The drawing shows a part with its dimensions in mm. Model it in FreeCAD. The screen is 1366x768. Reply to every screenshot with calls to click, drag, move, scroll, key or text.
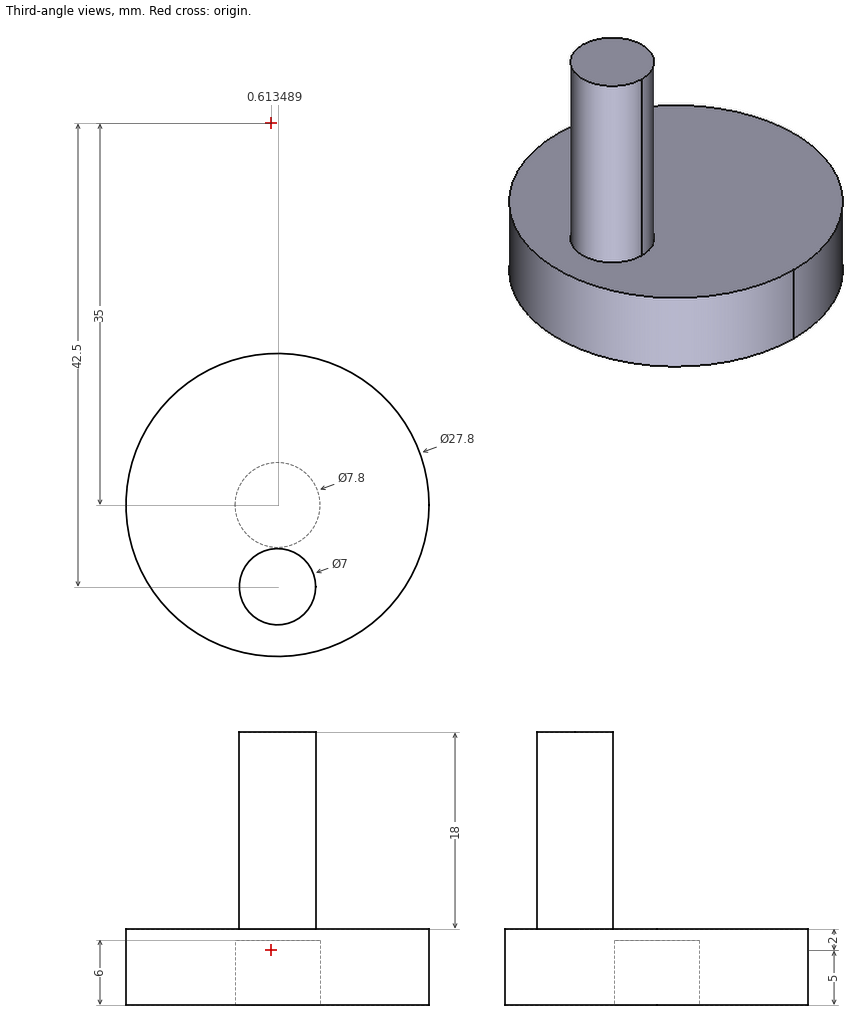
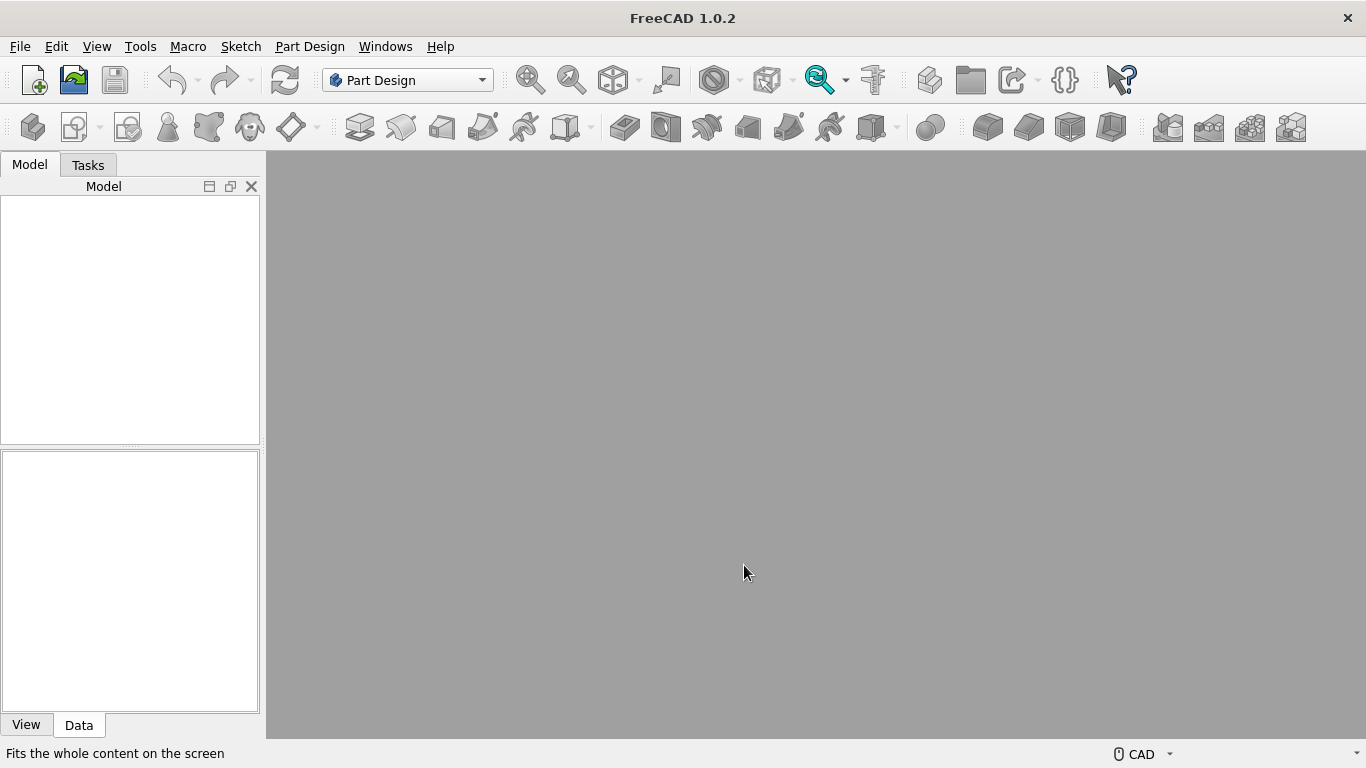
click(33, 80)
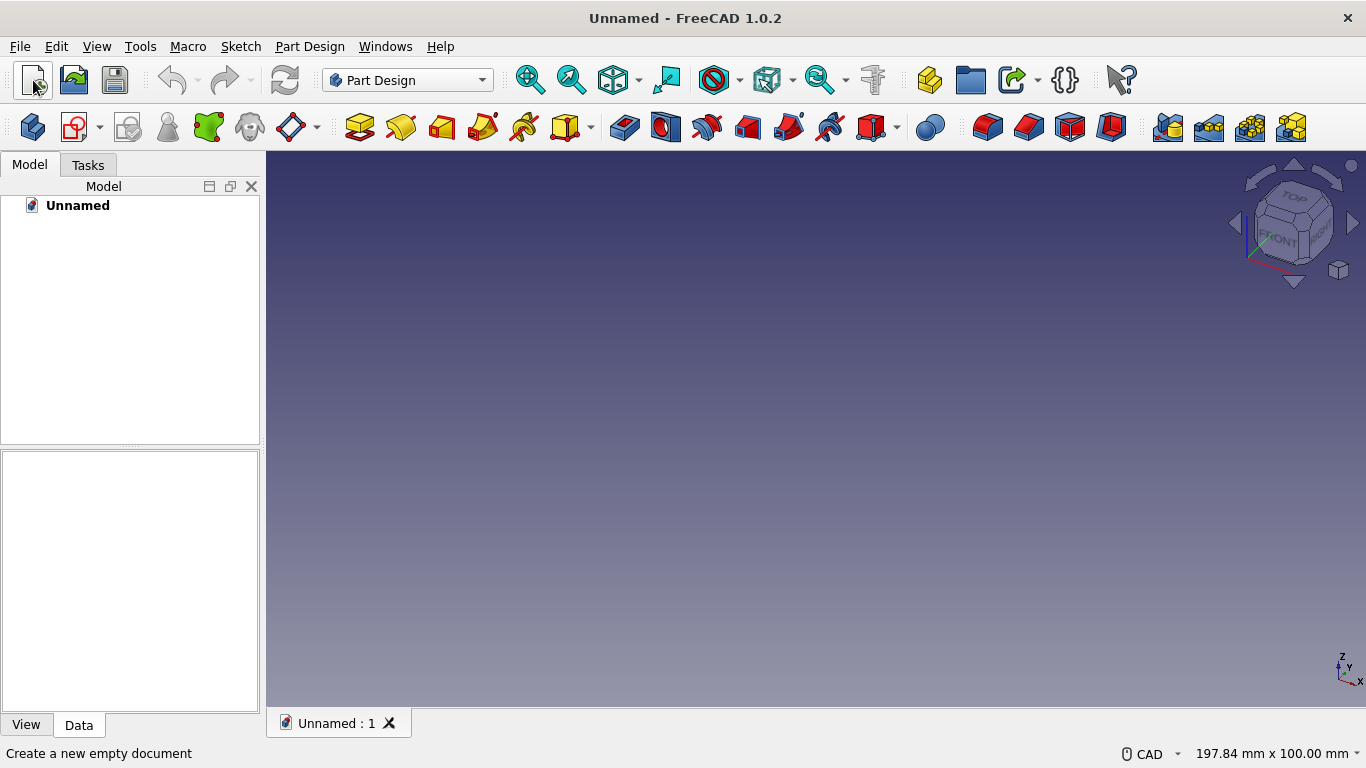
click(74, 128)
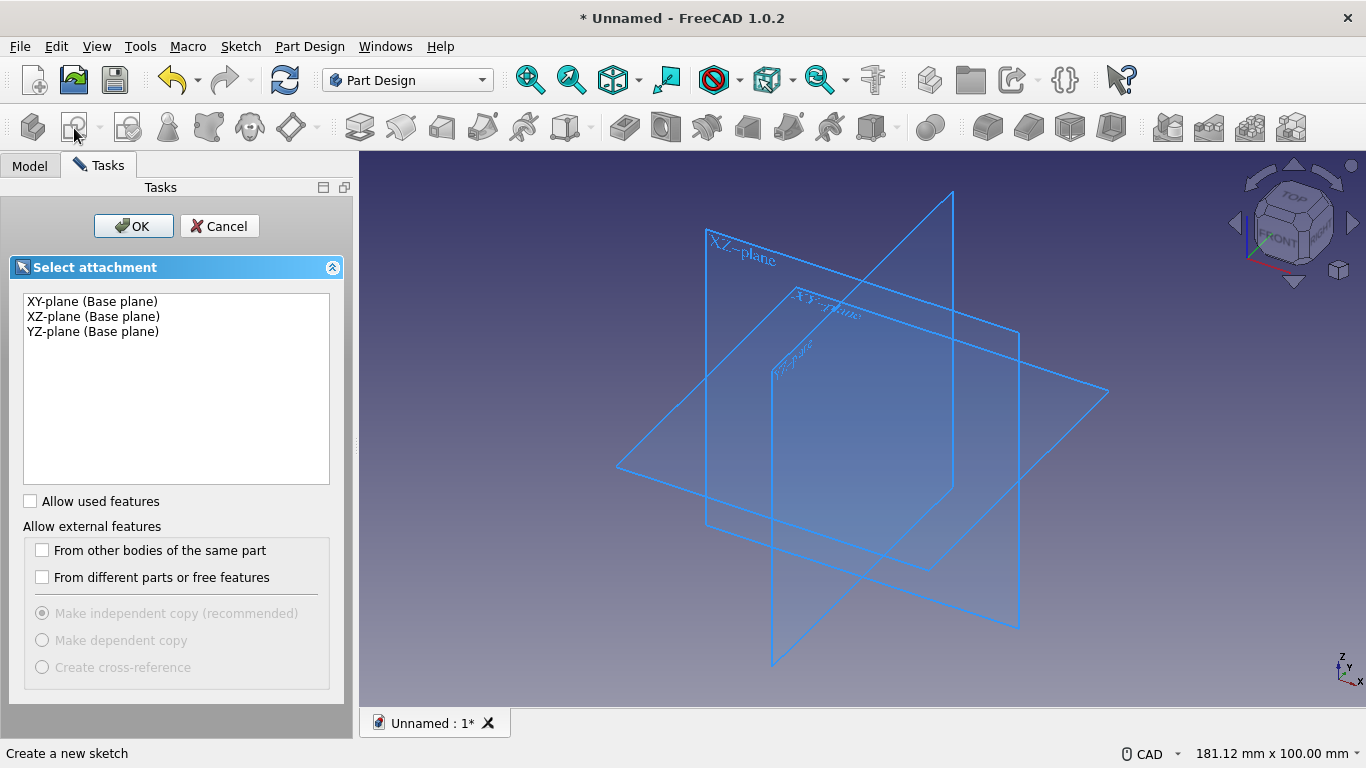
click(84, 302)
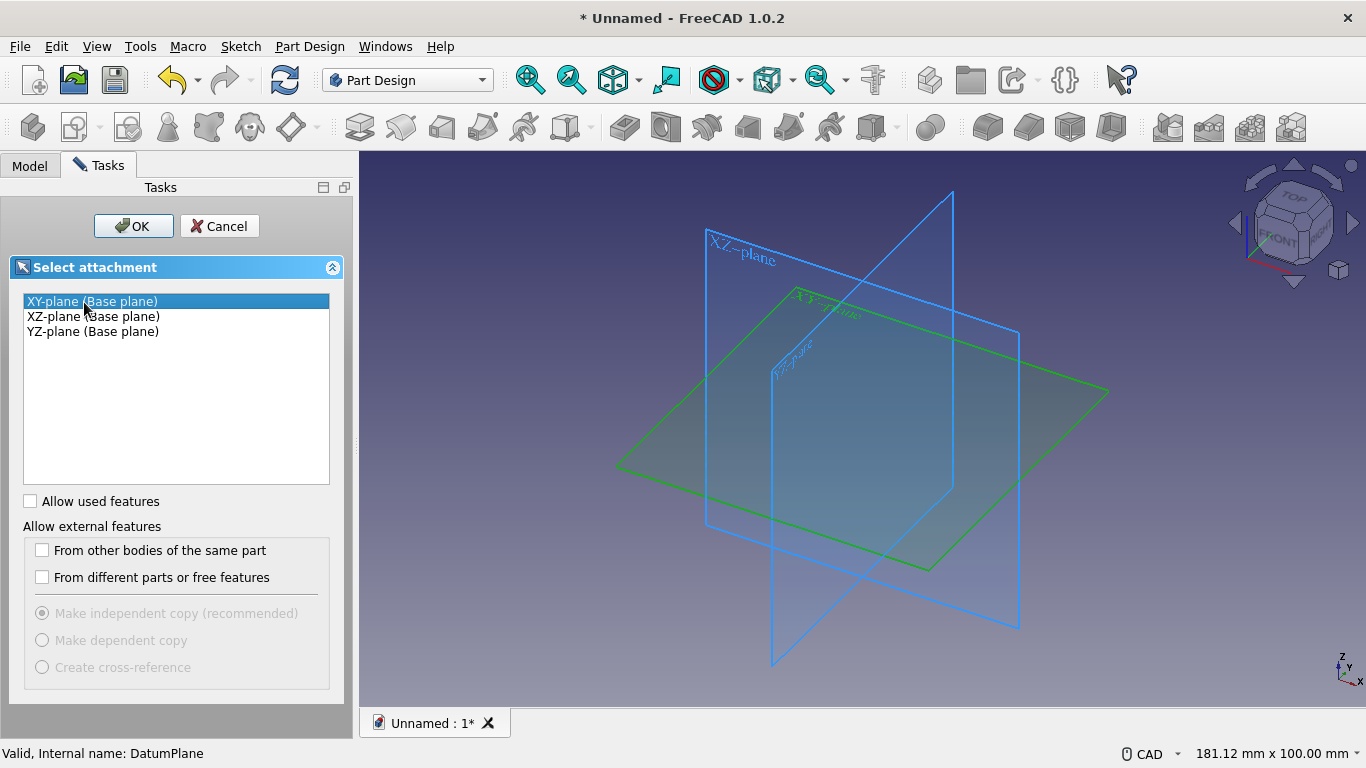
click(134, 226)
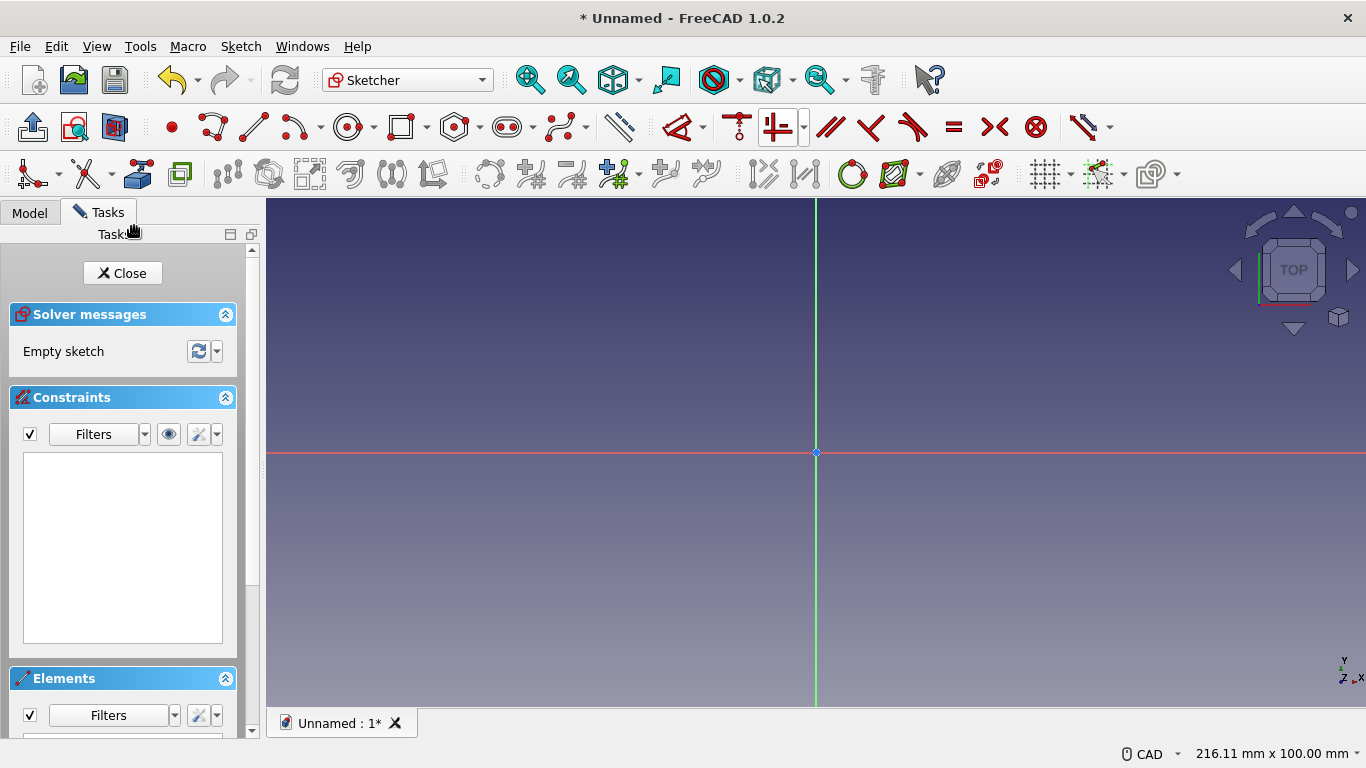
scroll(424, 226, down, 1)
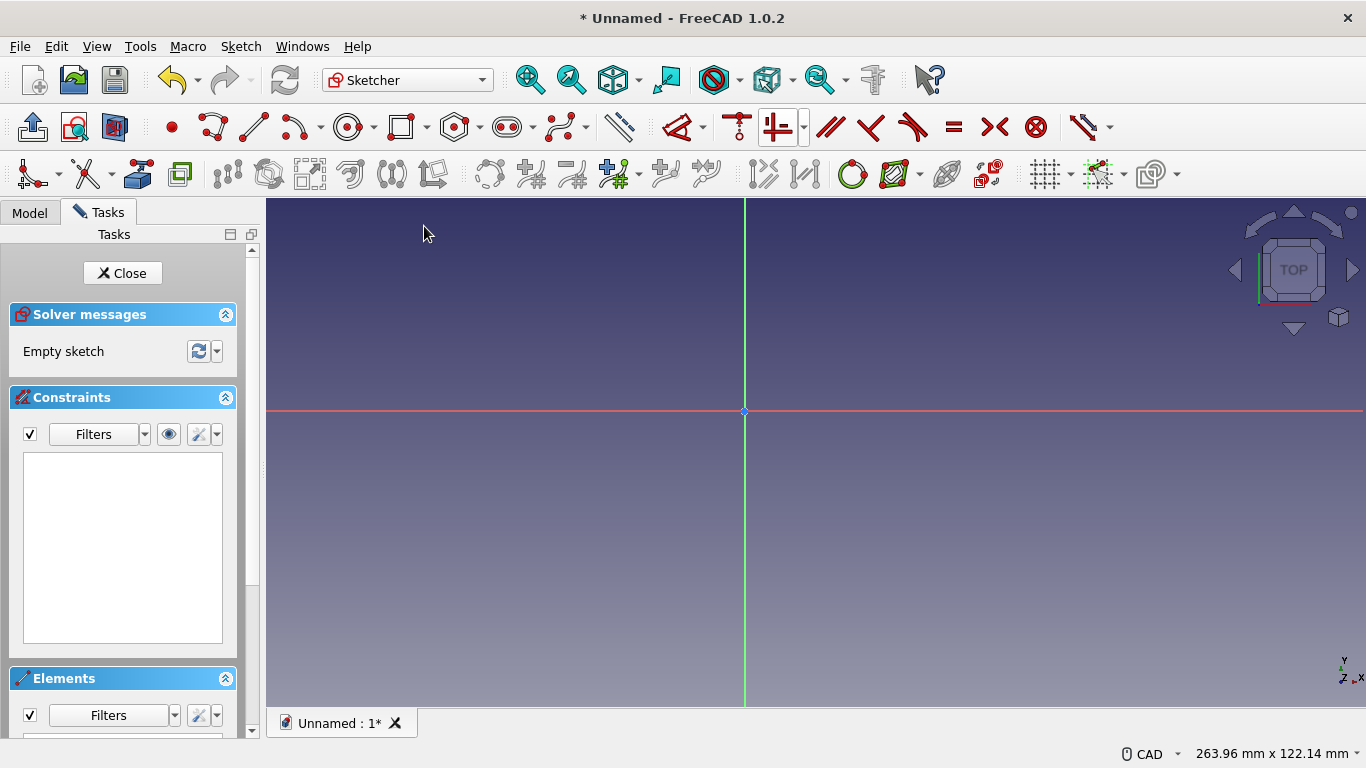
scroll(748, 637, up, 2)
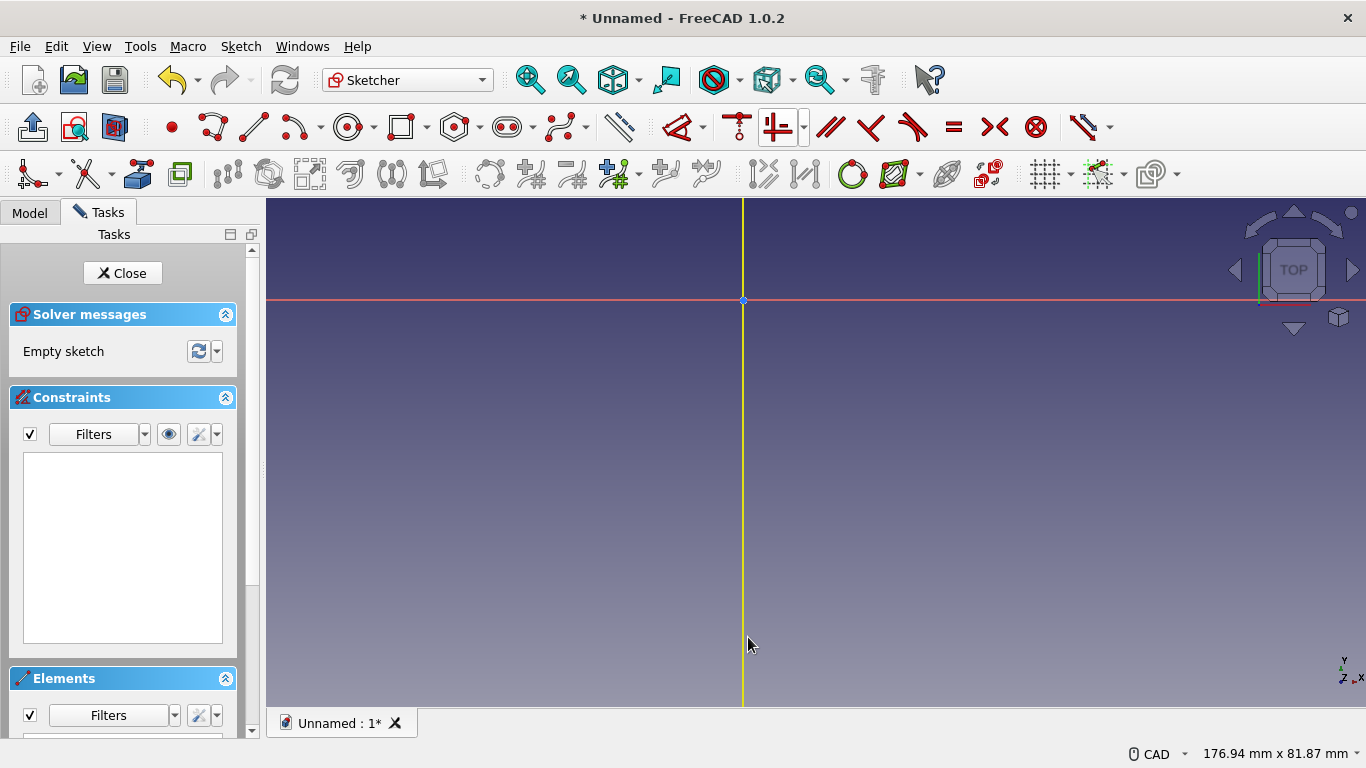
click(348, 128)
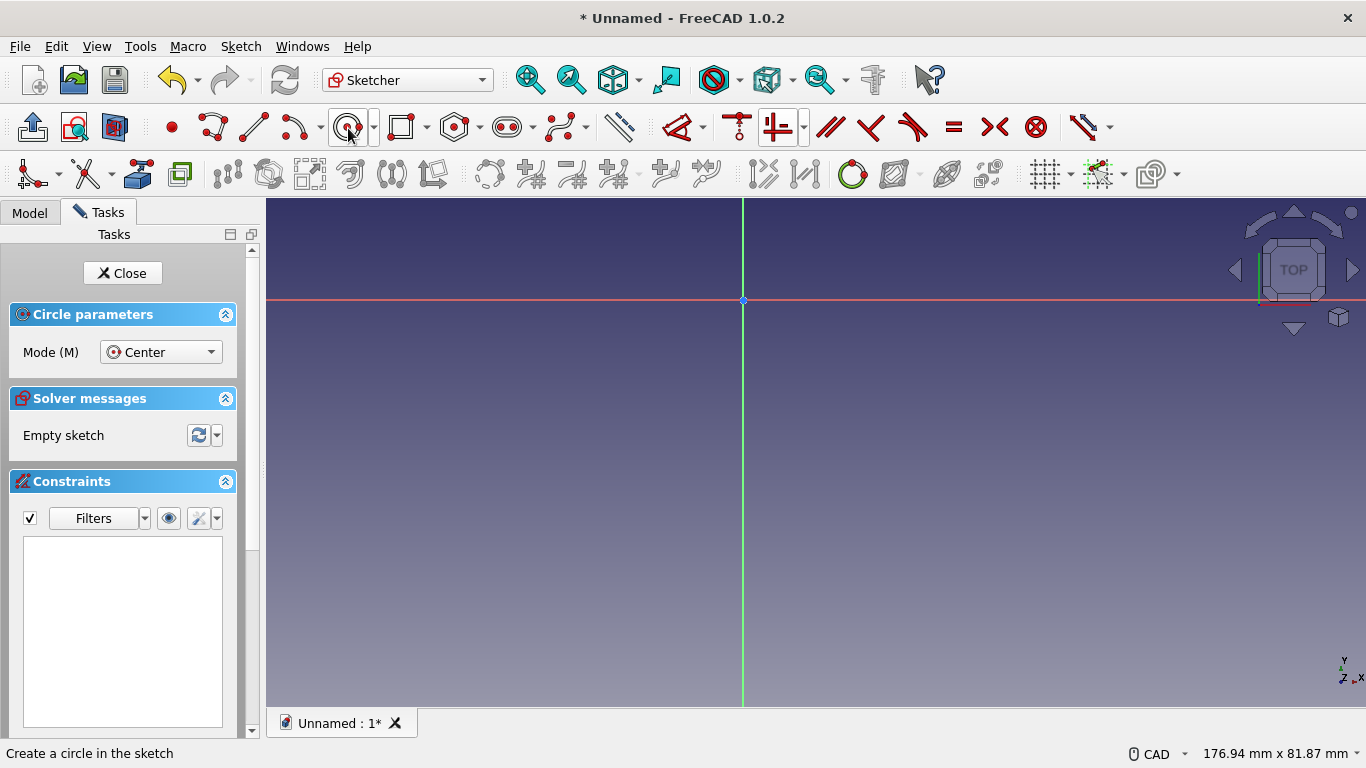
scroll(747, 518, up, 8)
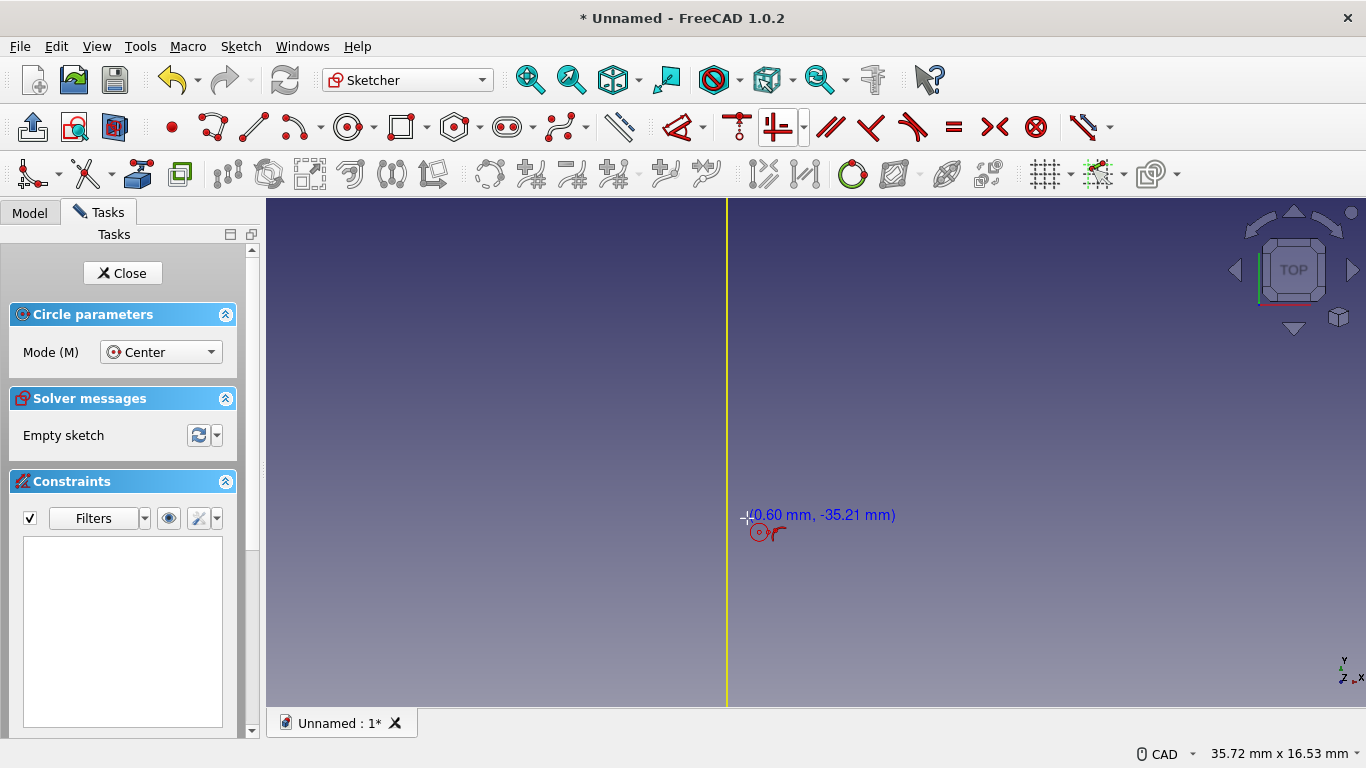
click(746, 514)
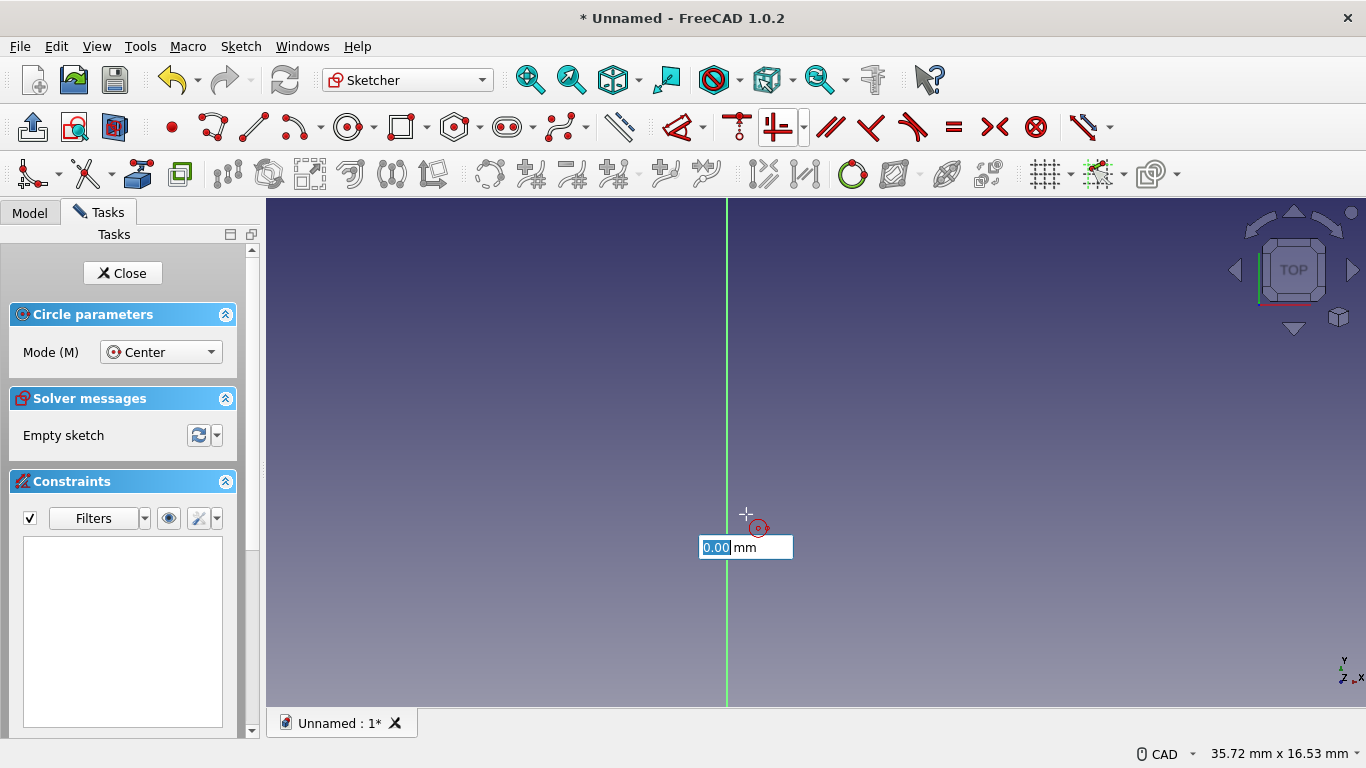
scroll(748, 519, down, 8)
move(809, 457)